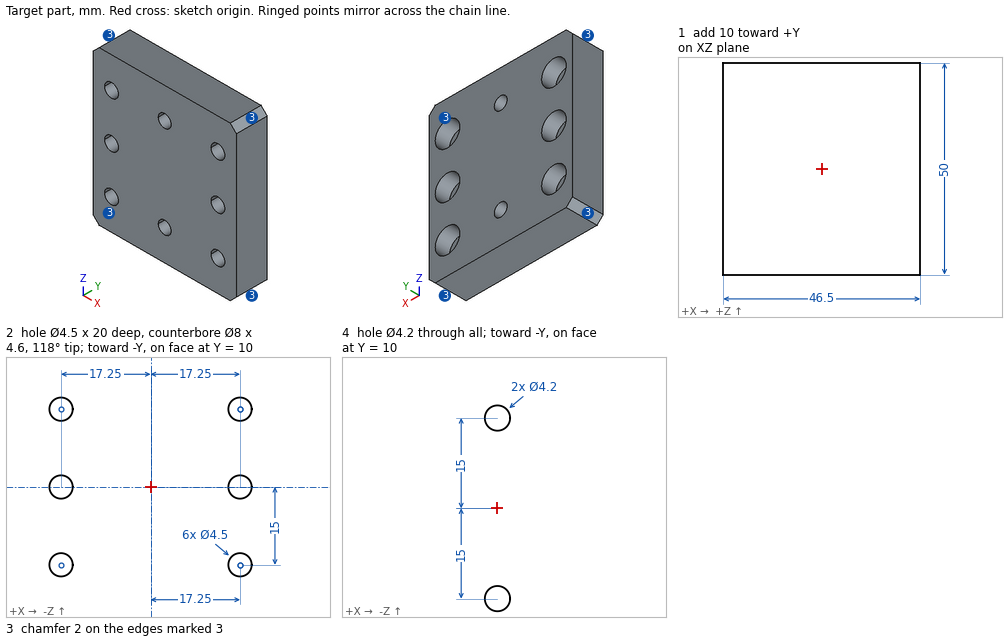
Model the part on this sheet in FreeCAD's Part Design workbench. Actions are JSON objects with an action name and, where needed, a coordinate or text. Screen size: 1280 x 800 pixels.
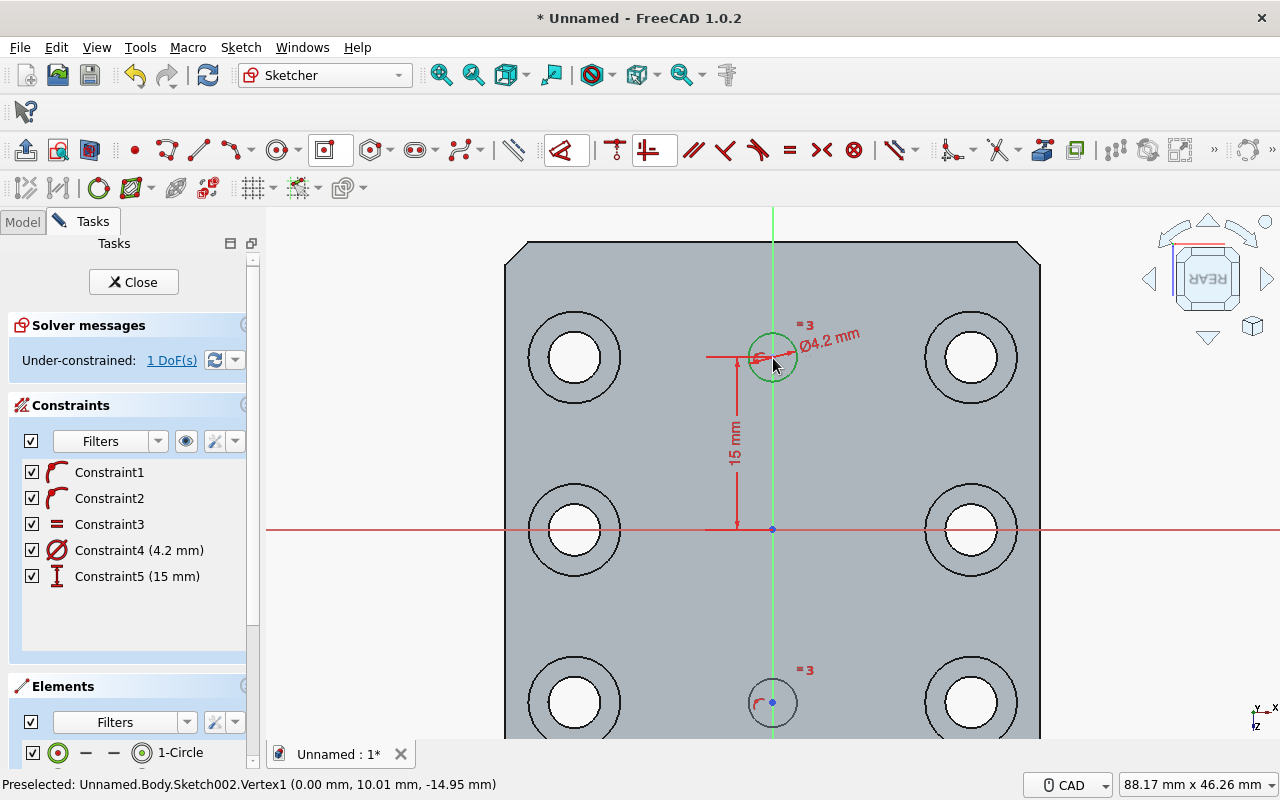
{"action": "left_click", "coordinate": [773, 703]}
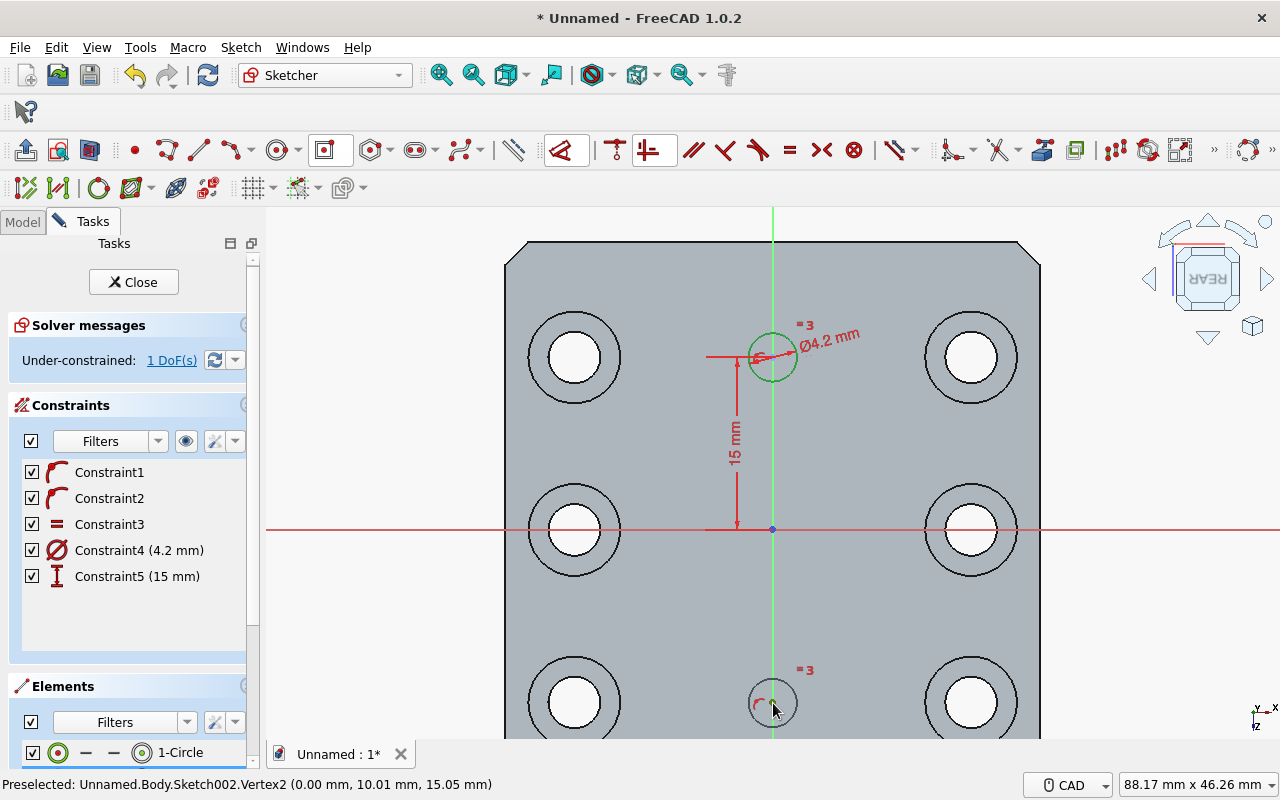
{"action": "left_click", "coordinate": [584, 150]}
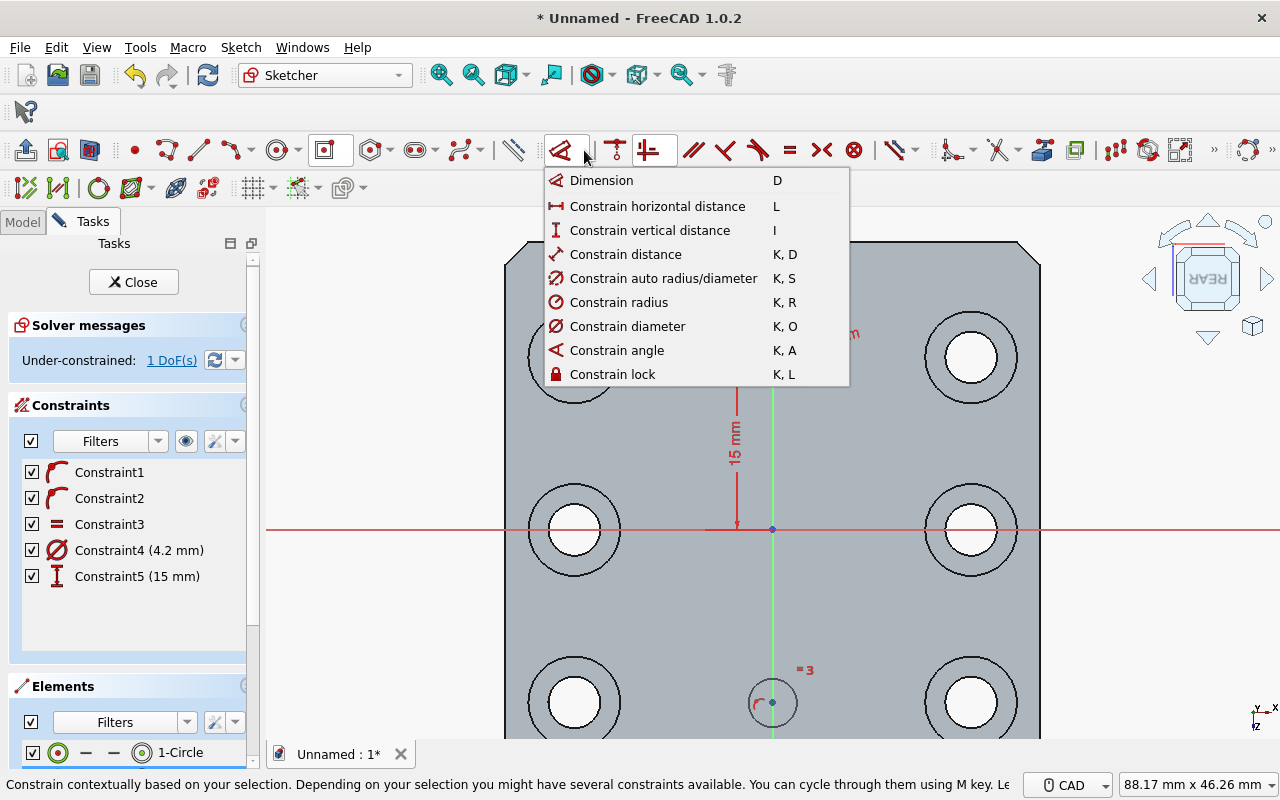
{"action": "left_click", "coordinate": [697, 230]}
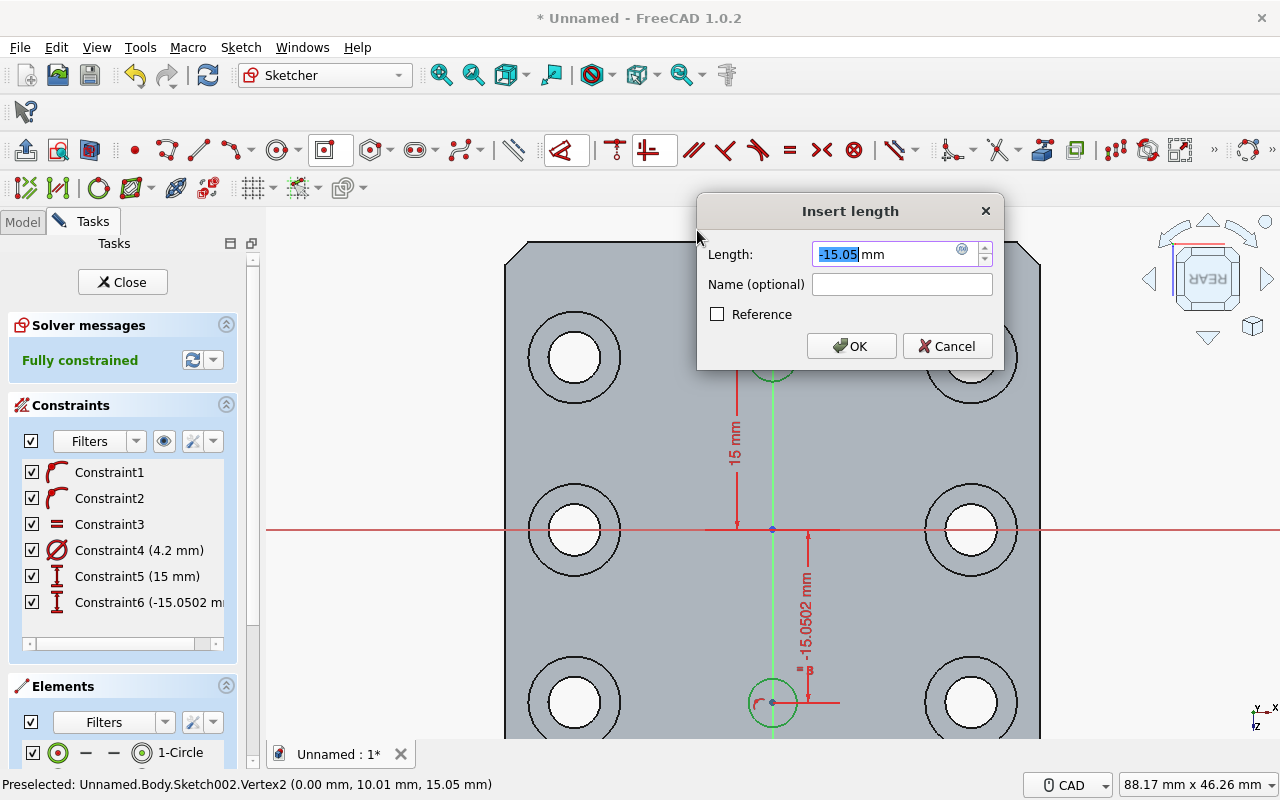
{"action": "type", "text": "-15"}
{"action": "key", "text": "Return"}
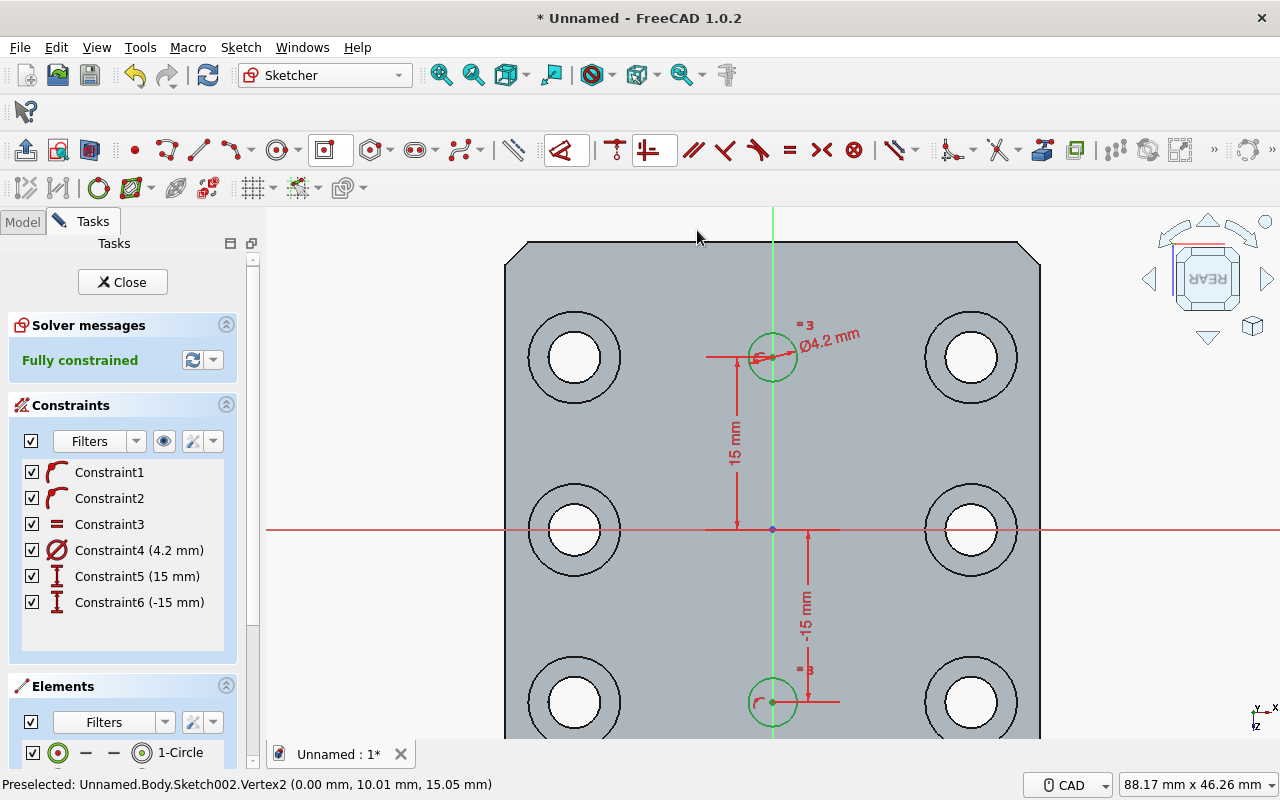
{"action": "left_click", "coordinate": [123, 282]}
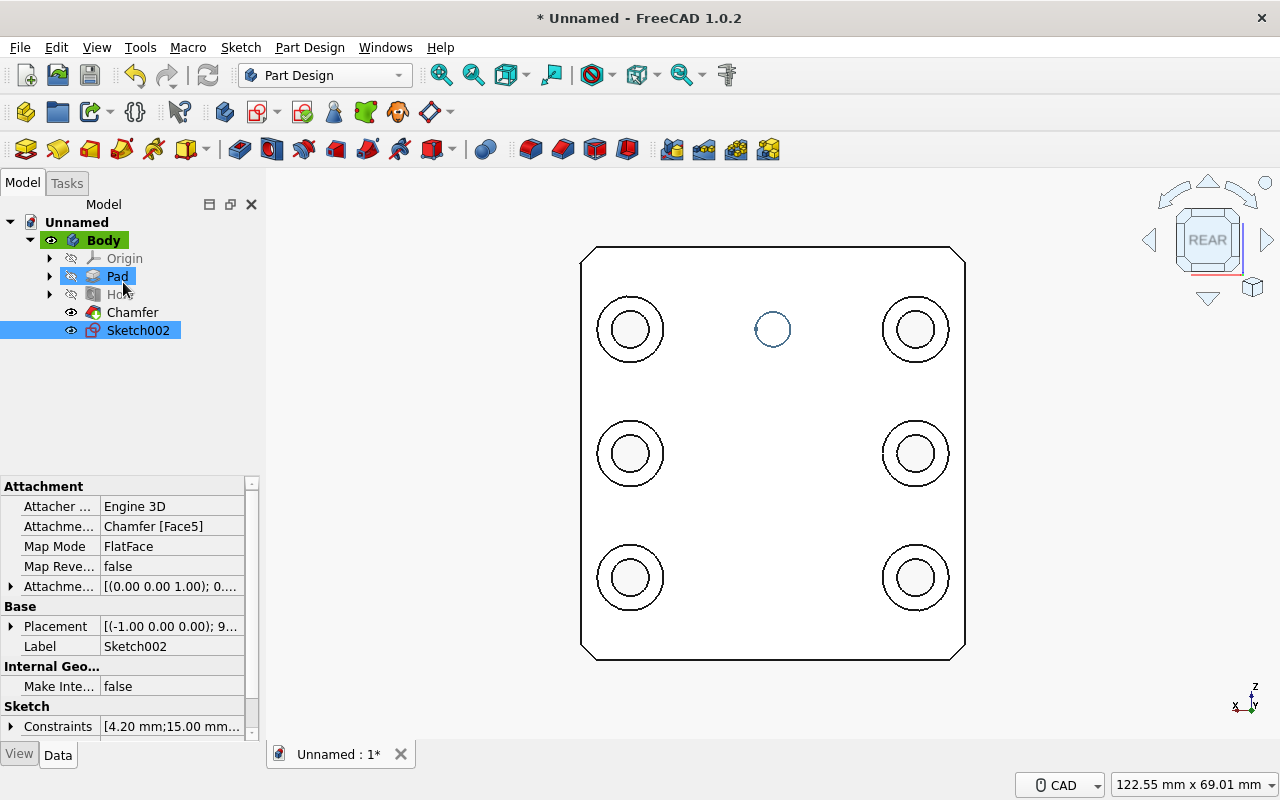
{"action": "left_click", "coordinate": [272, 150]}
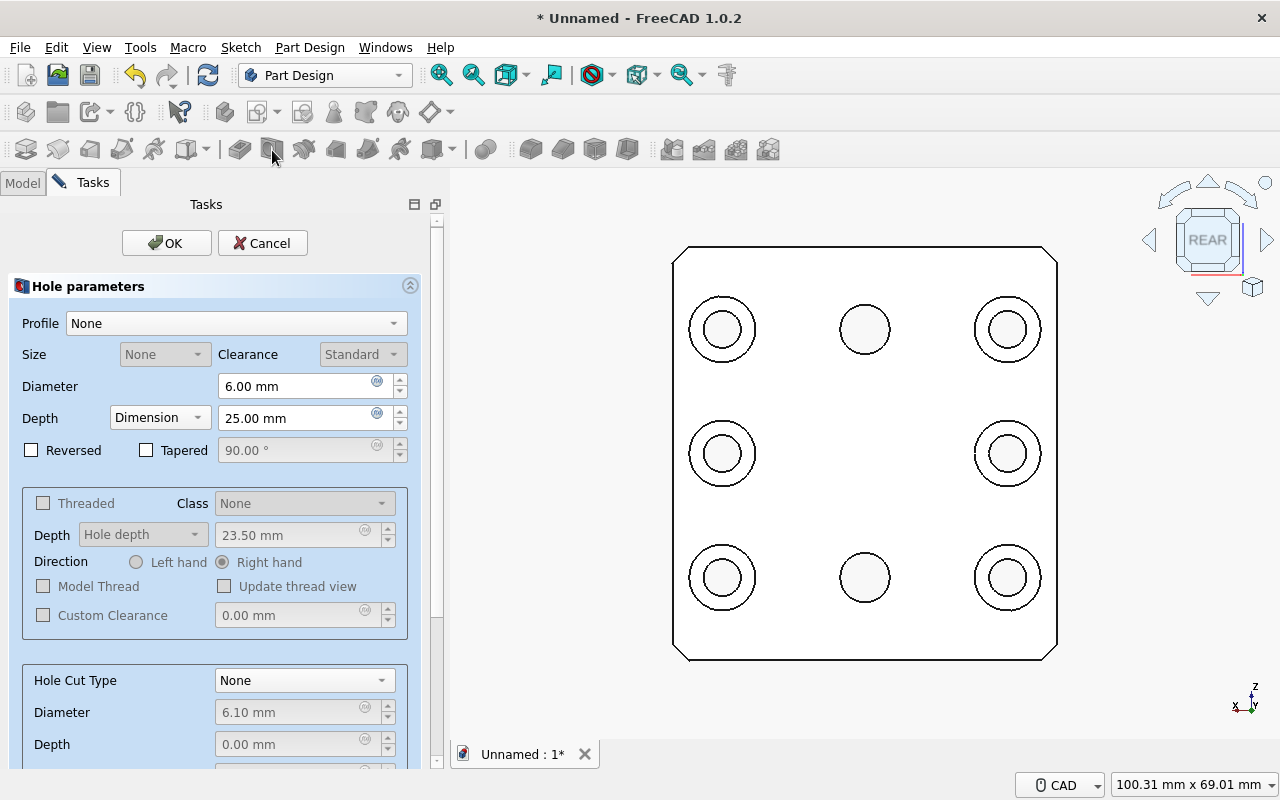
{"action": "triple_click", "coordinate": [305, 386]}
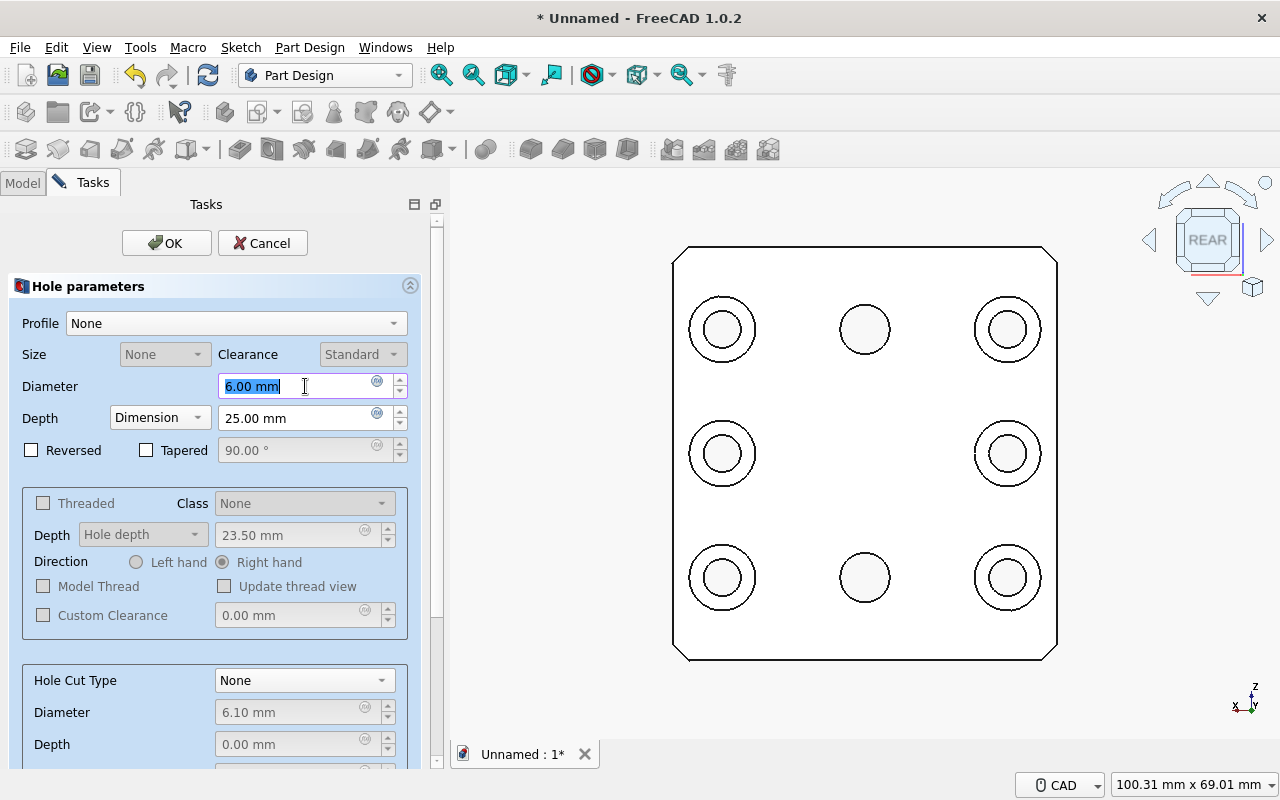
{"action": "type", "text": "4.2"}
{"action": "key", "text": "Tab"}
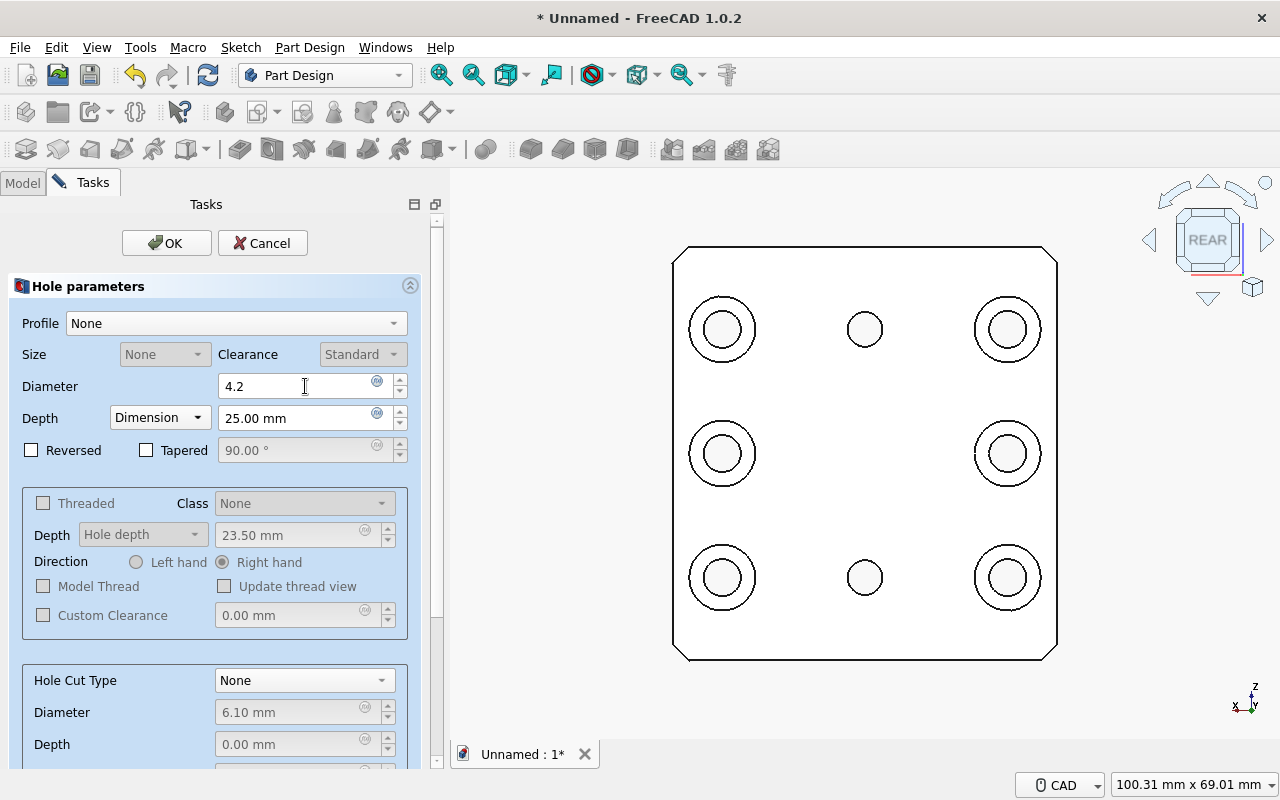
{"action": "left_click", "coordinate": [161, 418]}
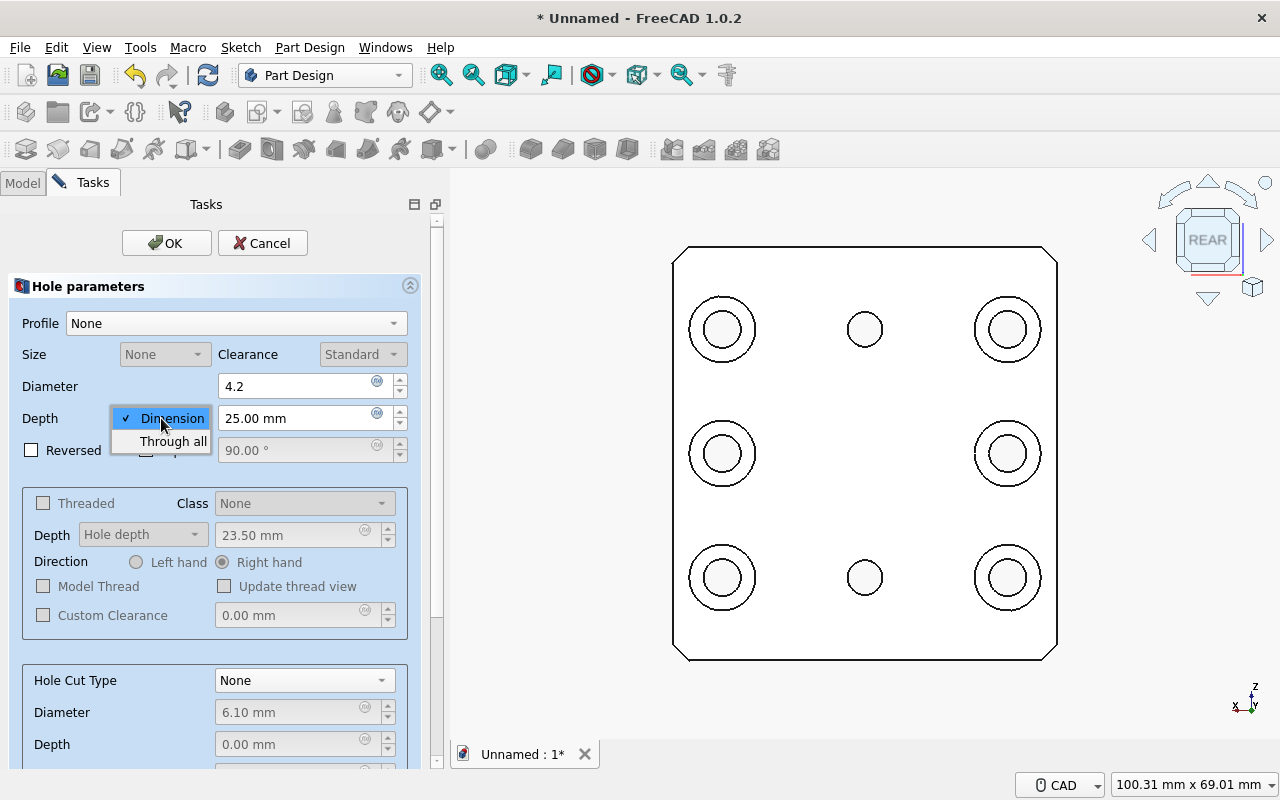
{"action": "left_click", "coordinate": [160, 442]}